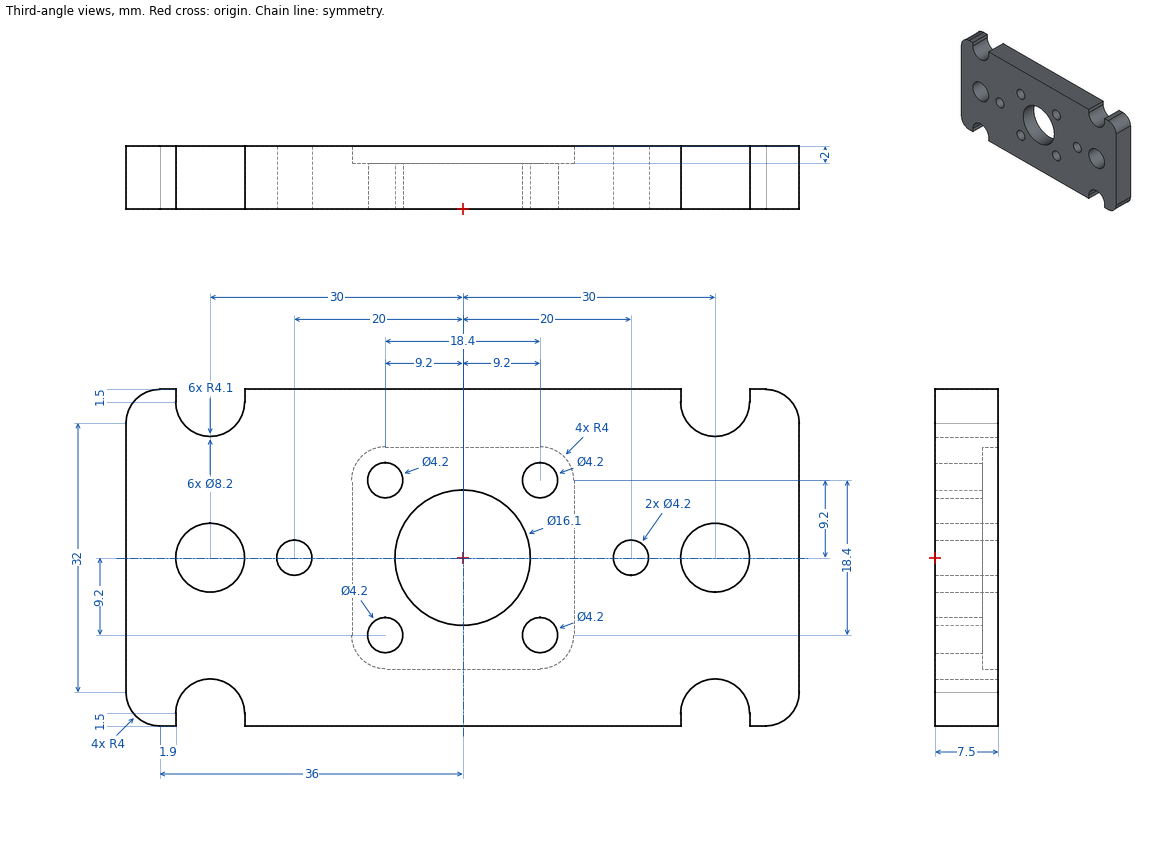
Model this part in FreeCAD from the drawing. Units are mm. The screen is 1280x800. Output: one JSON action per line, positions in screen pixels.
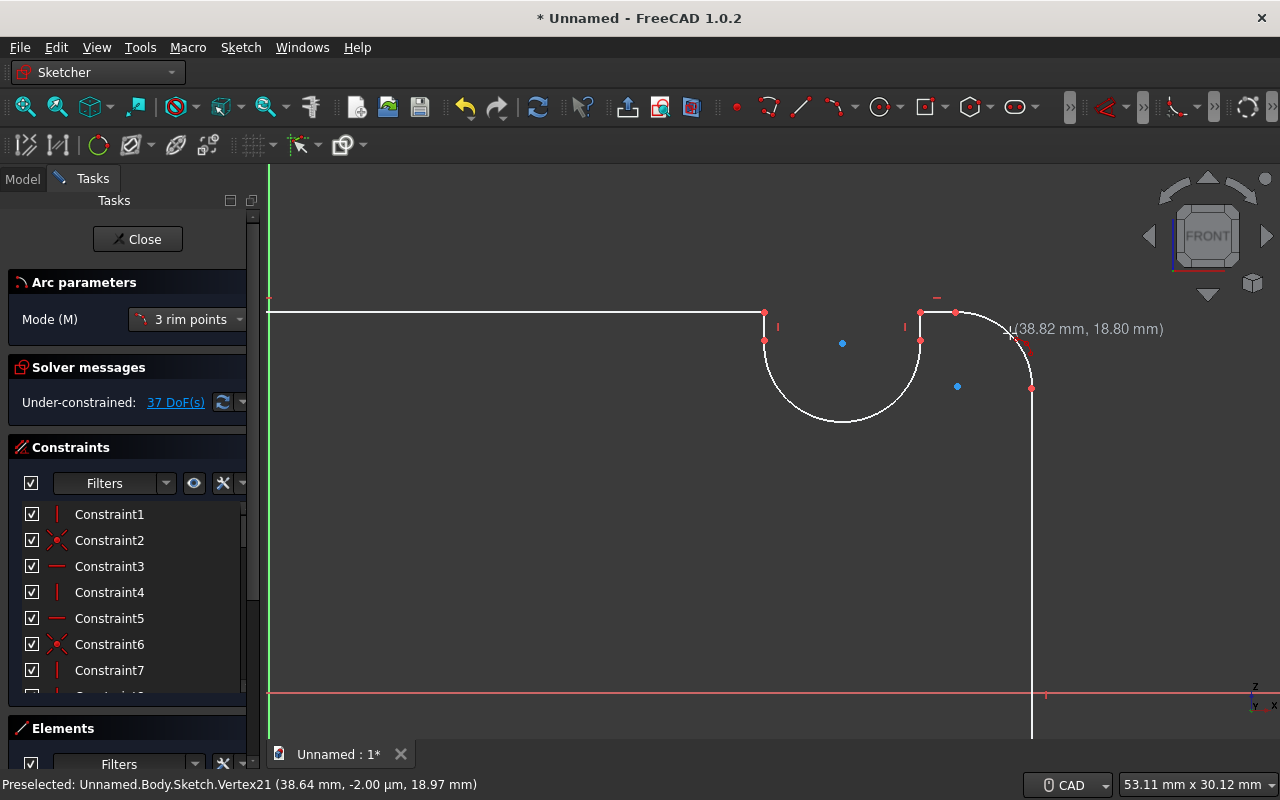
{"action": "scroll", "coordinate": [958, 311], "scroll_direction": "down", "scroll_amount": 5}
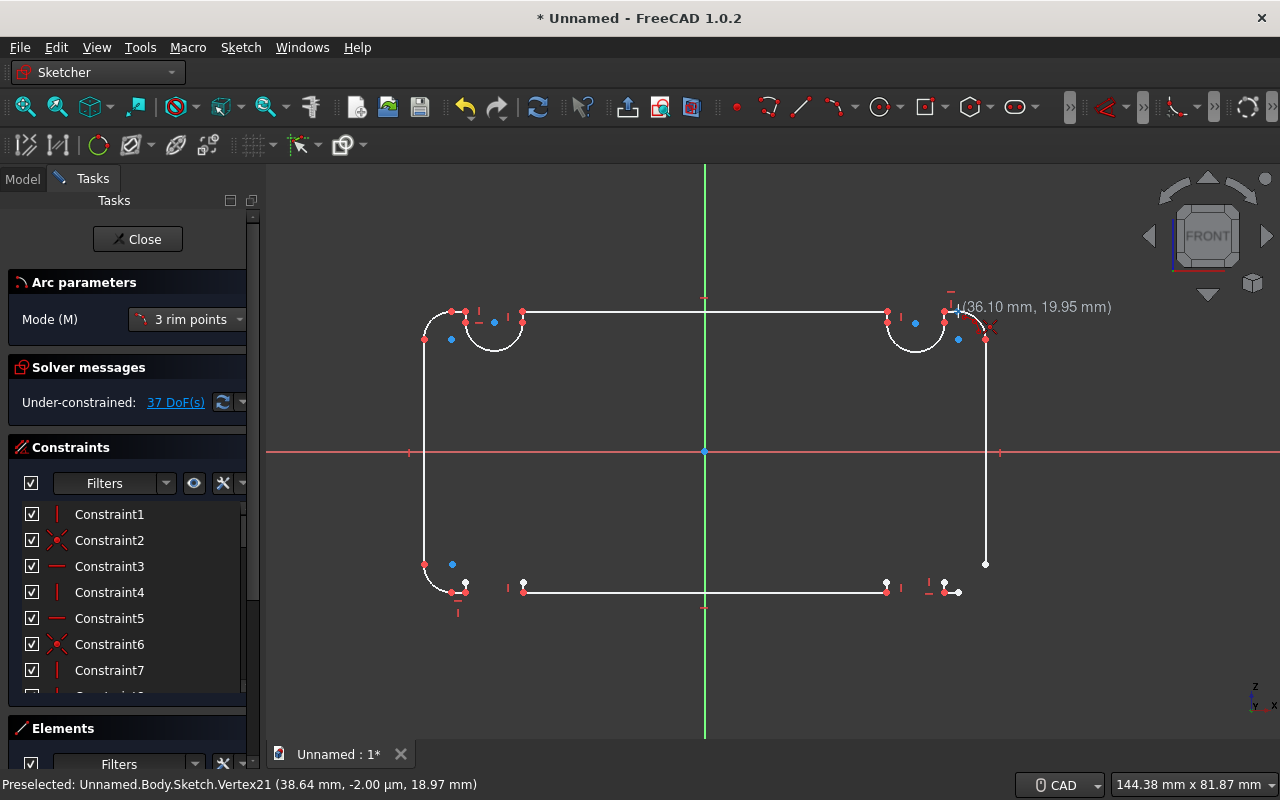
{"action": "left_click", "coordinate": [986, 565]}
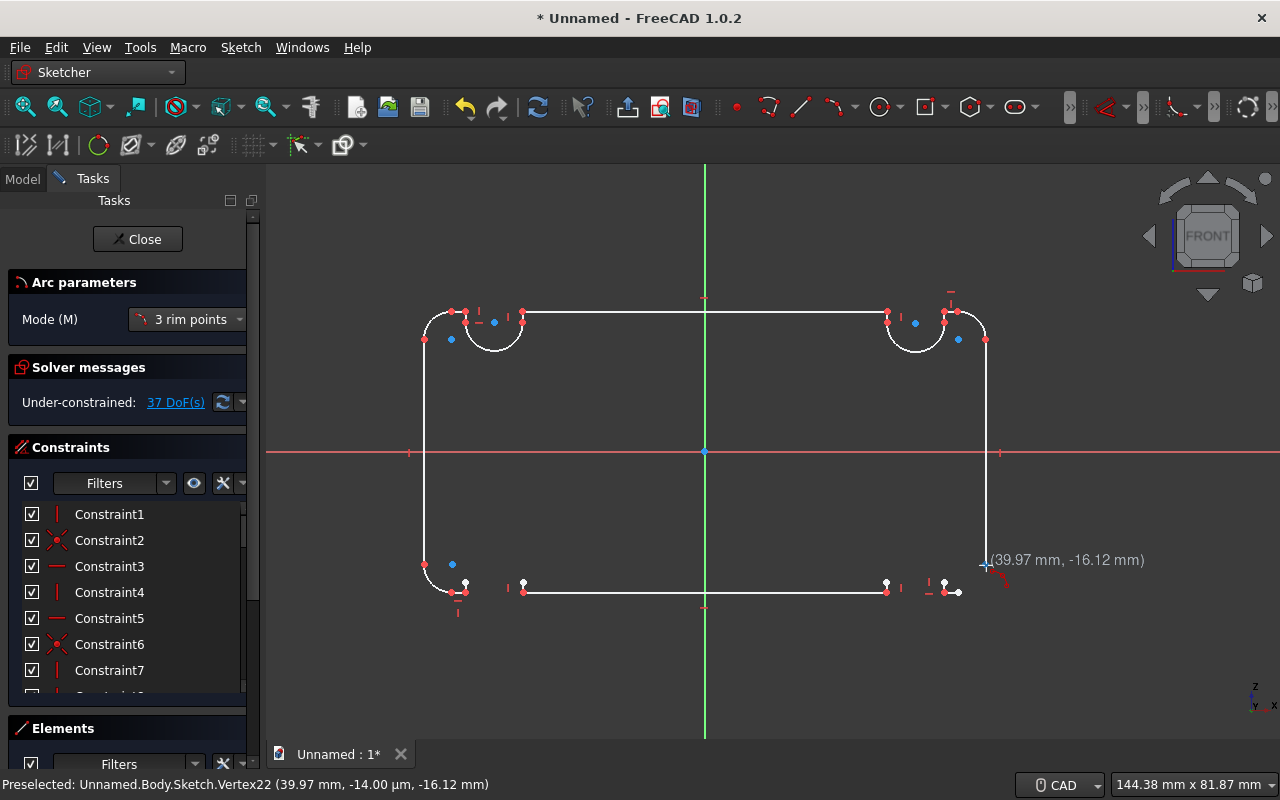
{"action": "scroll", "coordinate": [958, 592], "scroll_direction": "up", "scroll_amount": 5}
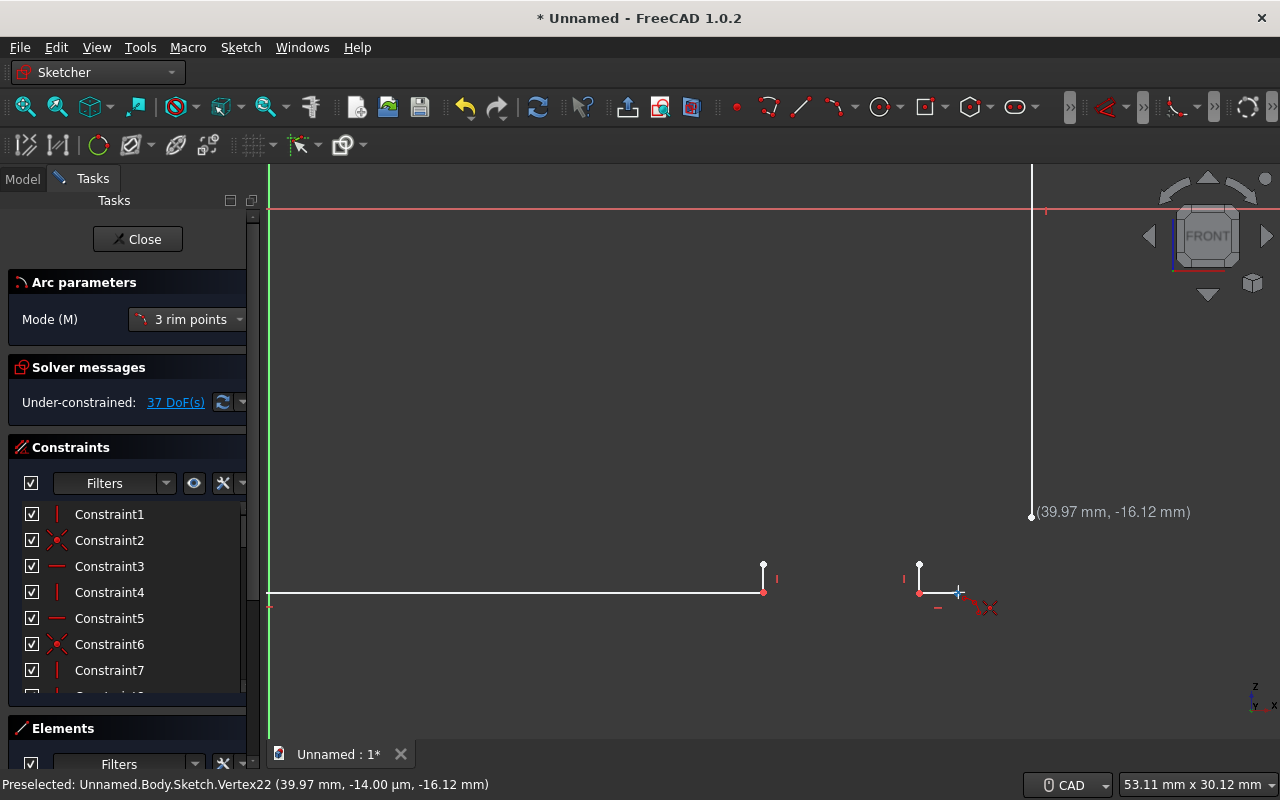
{"action": "left_click", "coordinate": [957, 593]}
{"action": "left_click", "coordinate": [1010, 569]}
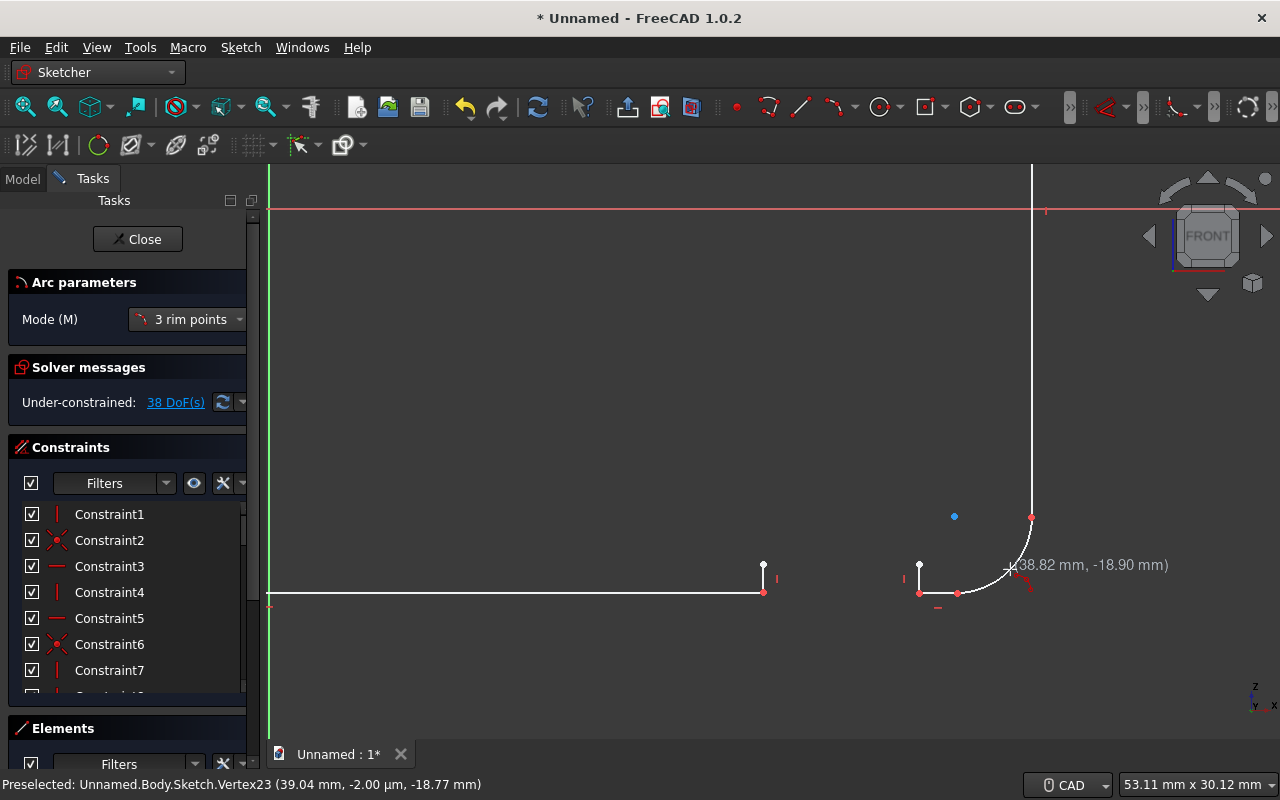
{"action": "left_click", "coordinate": [919, 564]}
{"action": "left_click", "coordinate": [763, 564]}
{"action": "left_click", "coordinate": [842, 484]}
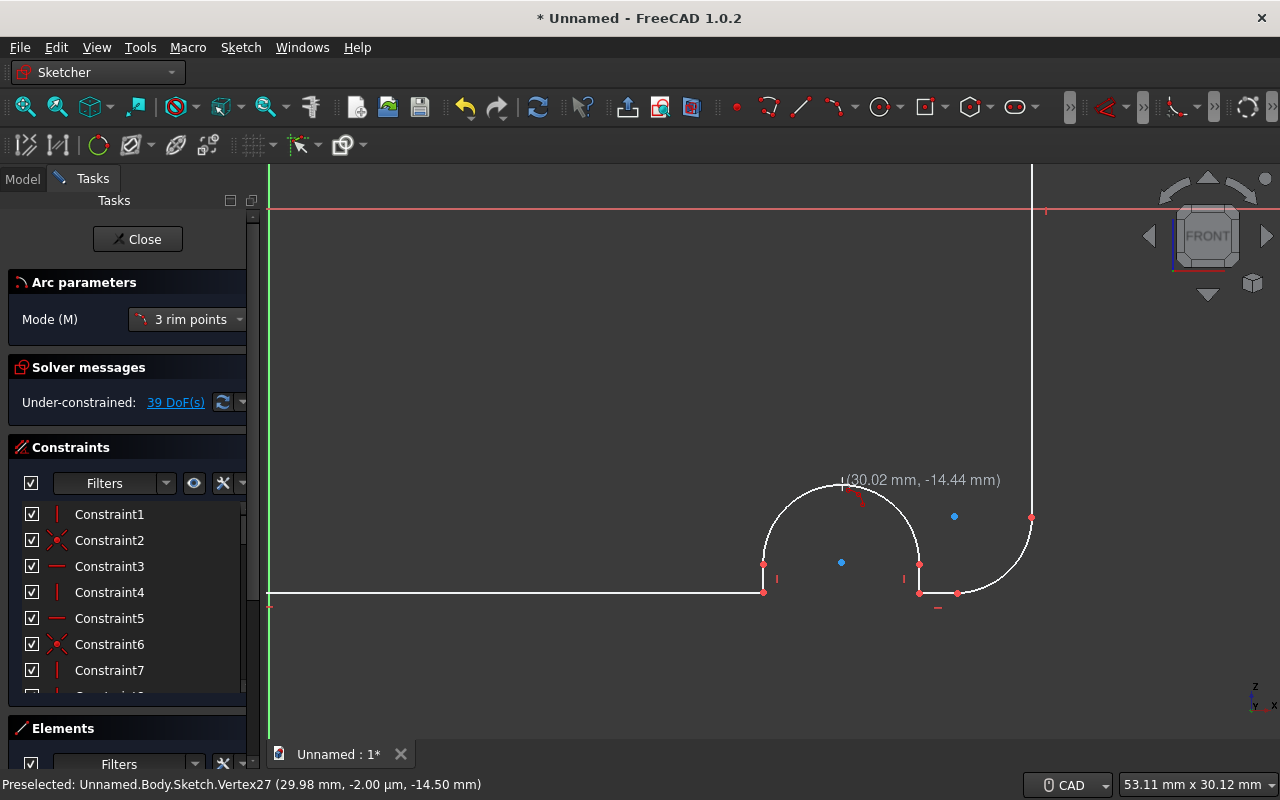
{"action": "scroll", "coordinate": [958, 592], "scroll_direction": "down", "scroll_amount": 5}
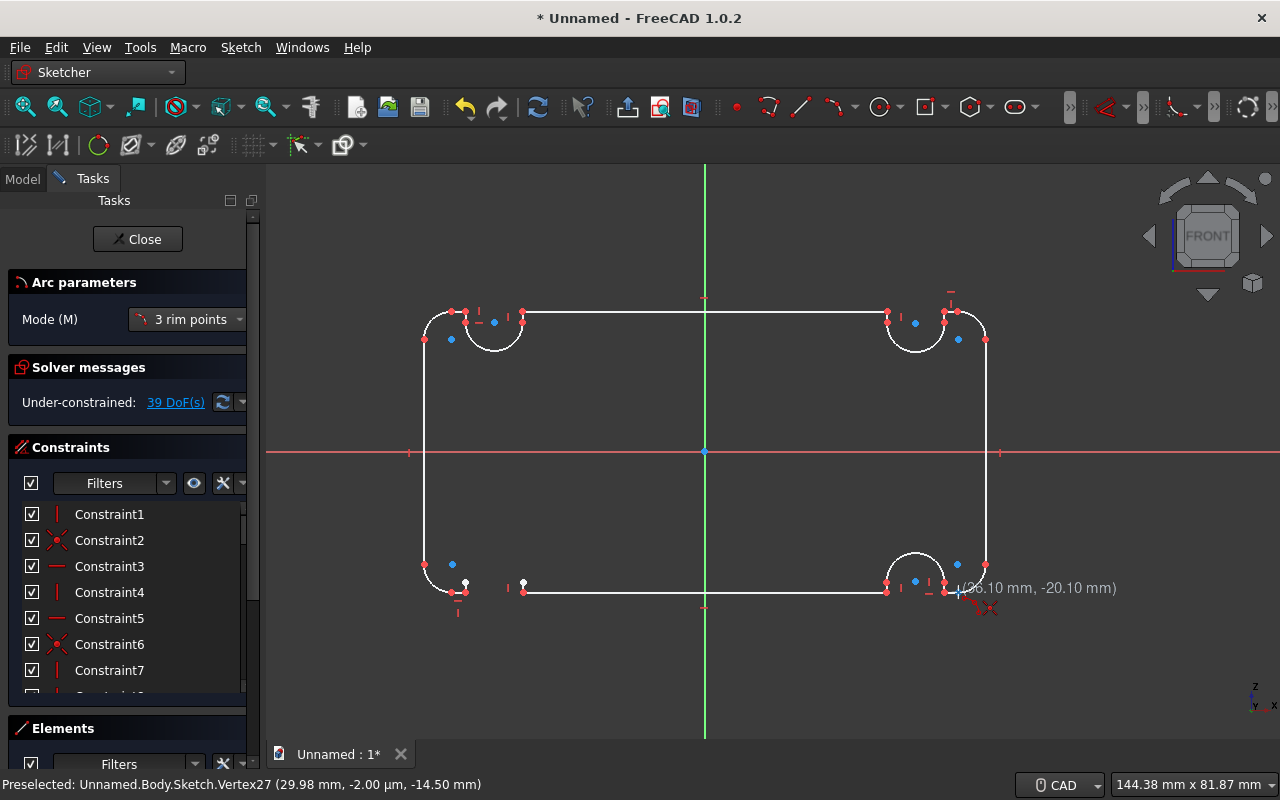
{"action": "scroll", "coordinate": [523, 582], "scroll_direction": "up", "scroll_amount": 6}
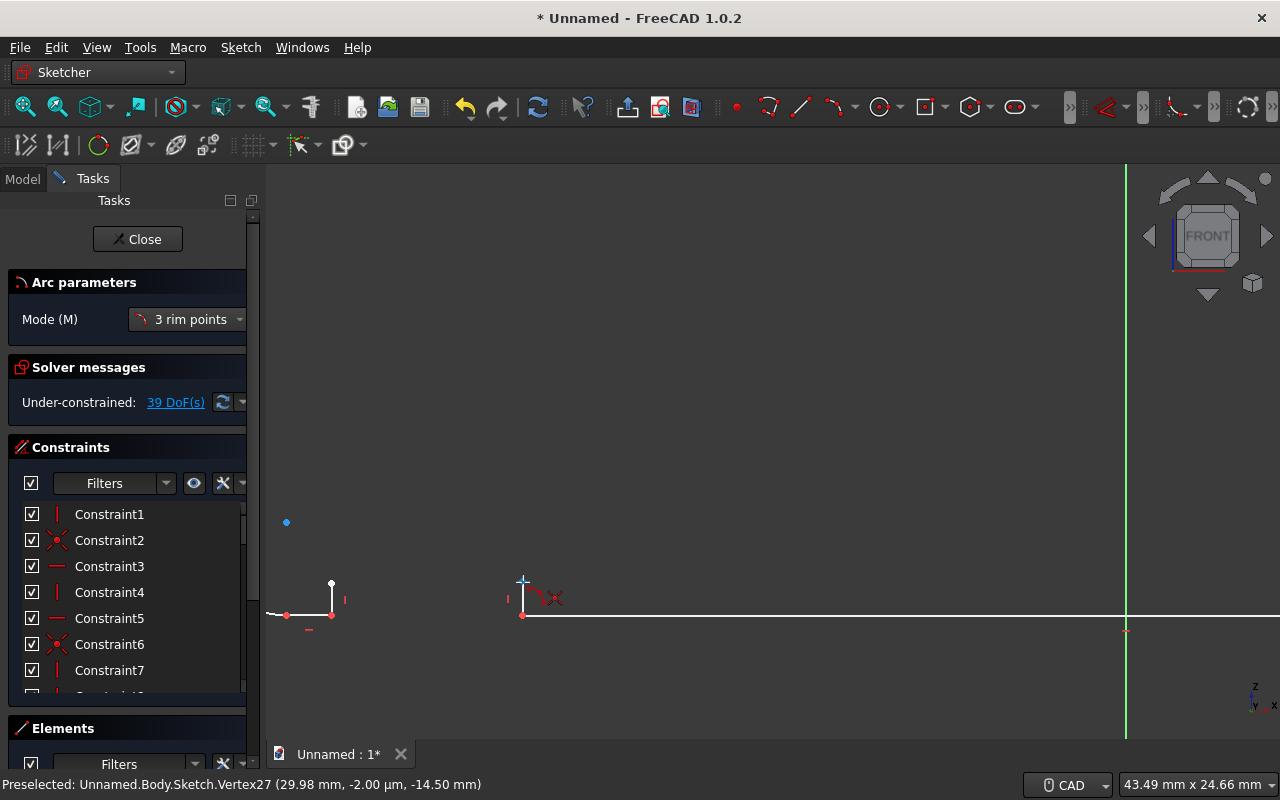
{"action": "left_click", "coordinate": [523, 581]}
{"action": "left_click", "coordinate": [332, 584]}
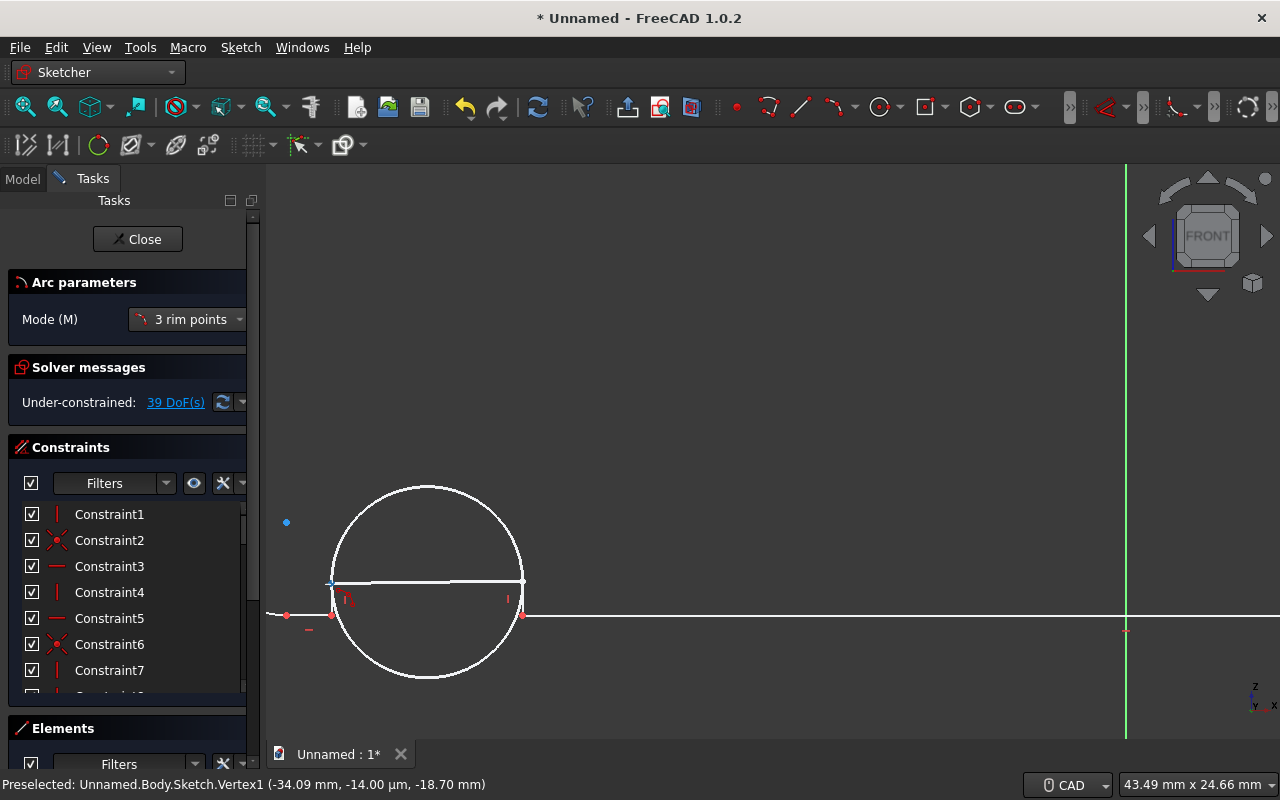
{"action": "scroll", "coordinate": [523, 582], "scroll_direction": "down", "scroll_amount": 6}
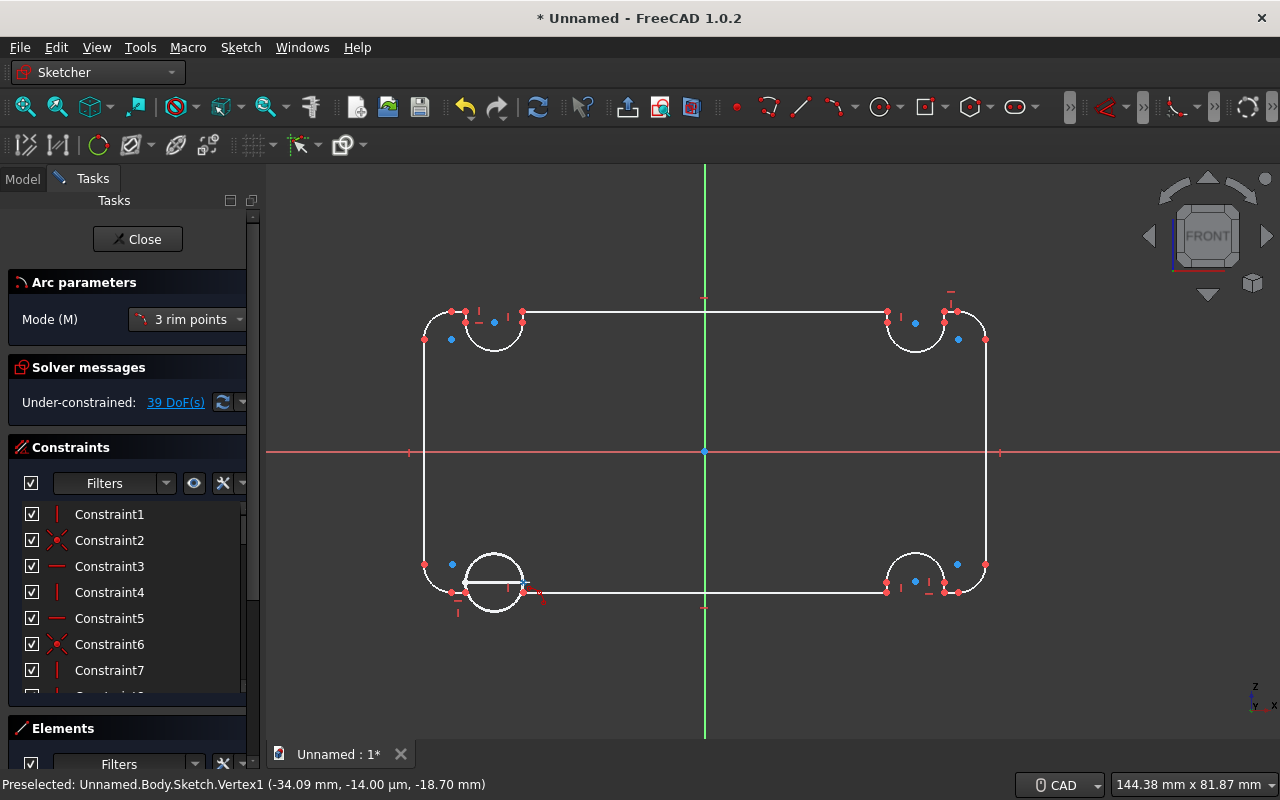
{"action": "left_click", "coordinate": [494, 553]}